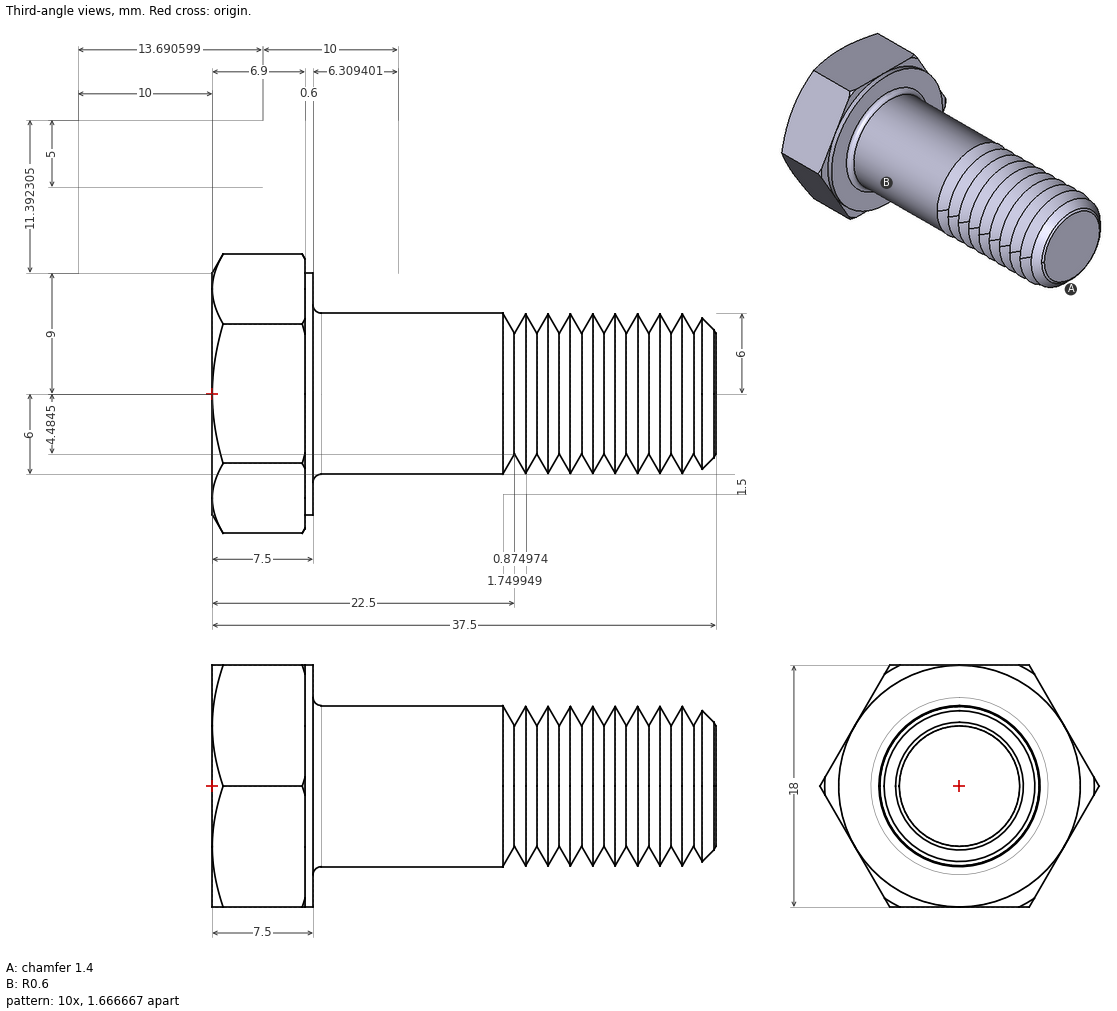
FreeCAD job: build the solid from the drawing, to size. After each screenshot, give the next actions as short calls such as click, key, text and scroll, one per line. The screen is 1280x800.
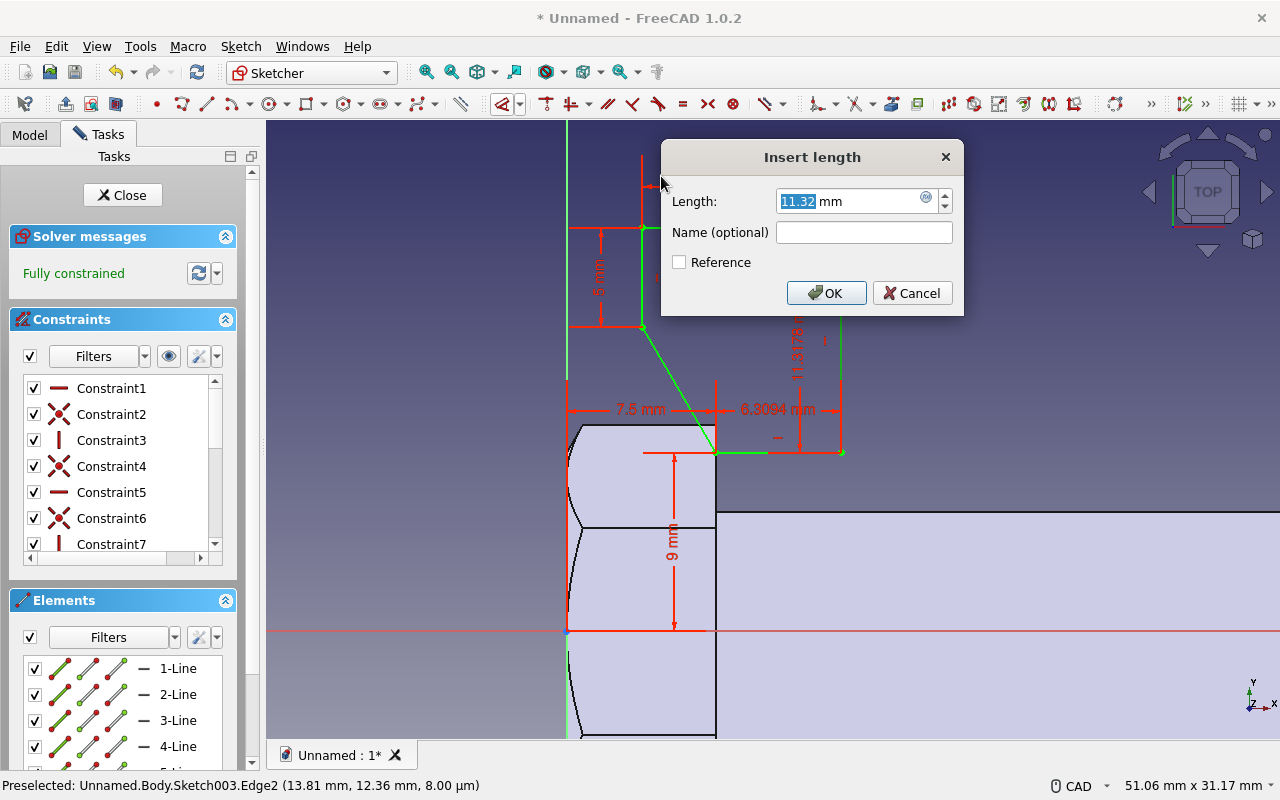
text(11.392305)
key(Return)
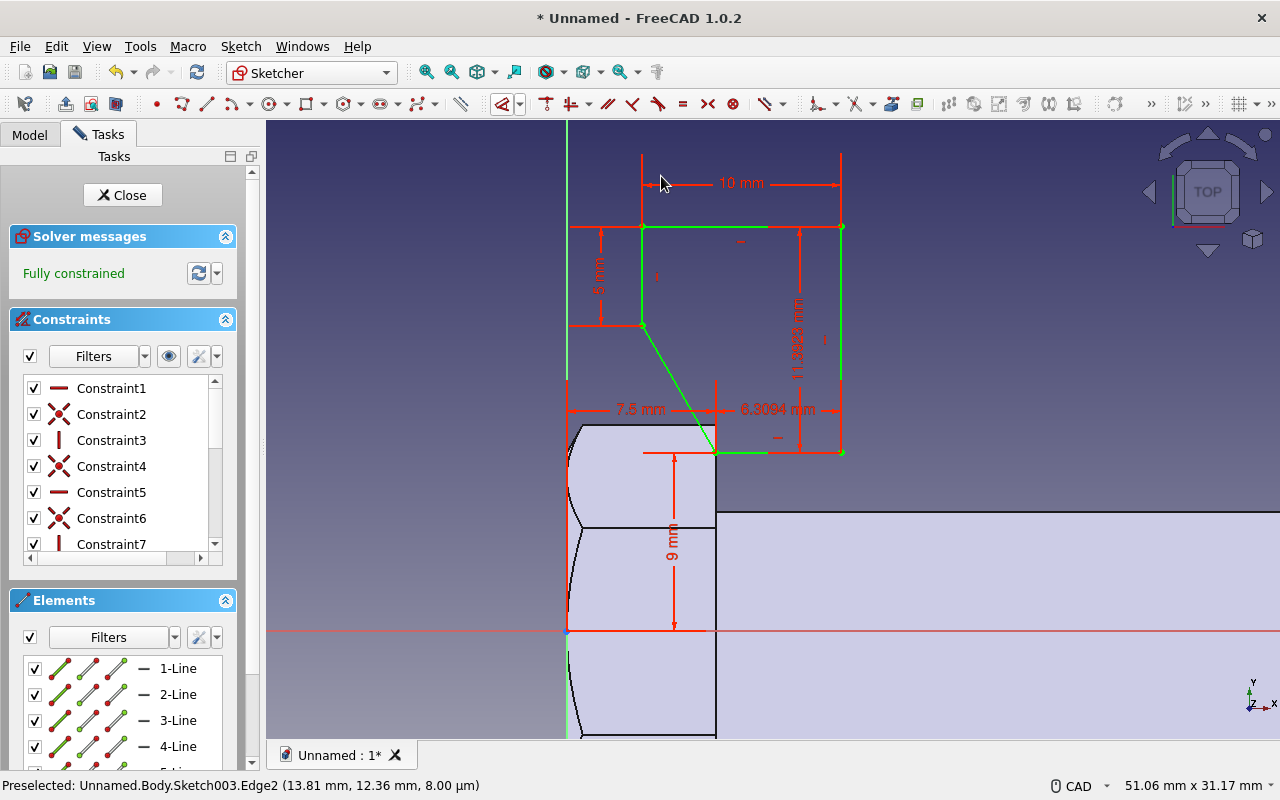
click(123, 195)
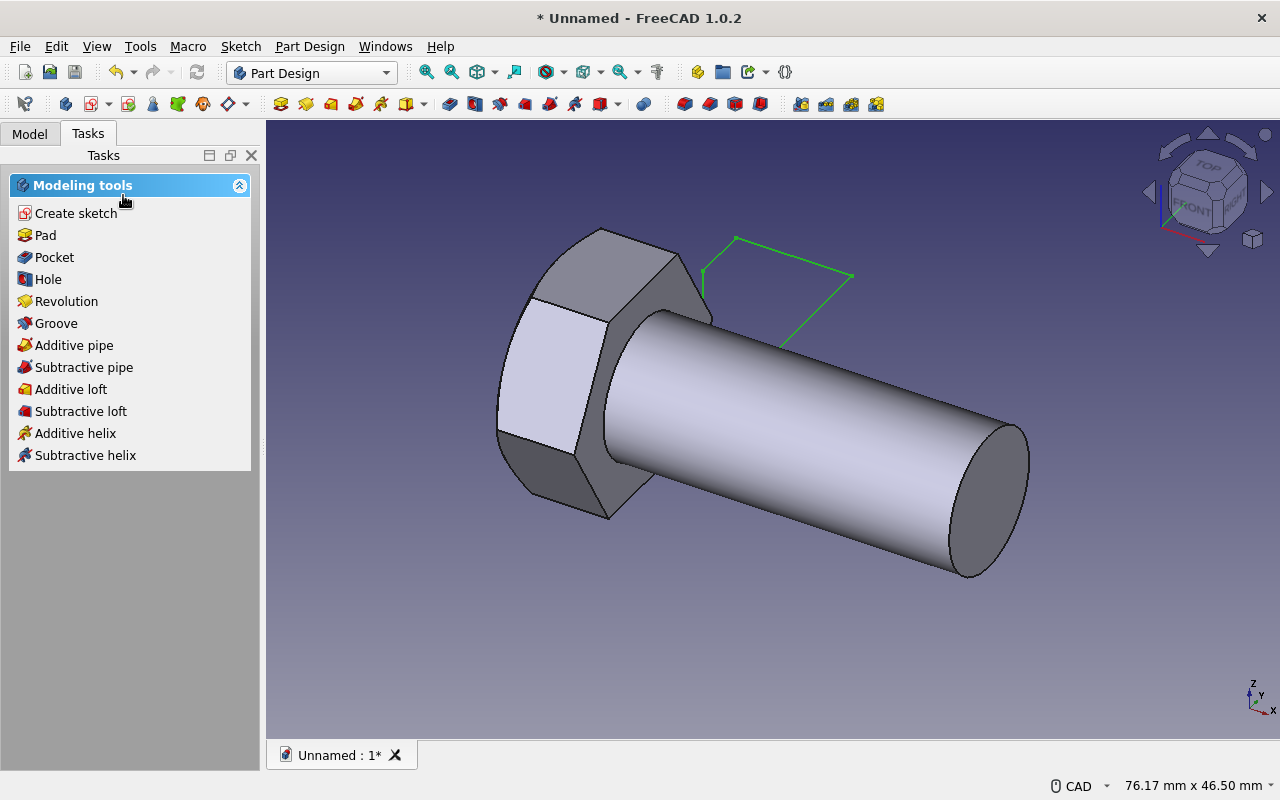
click(500, 104)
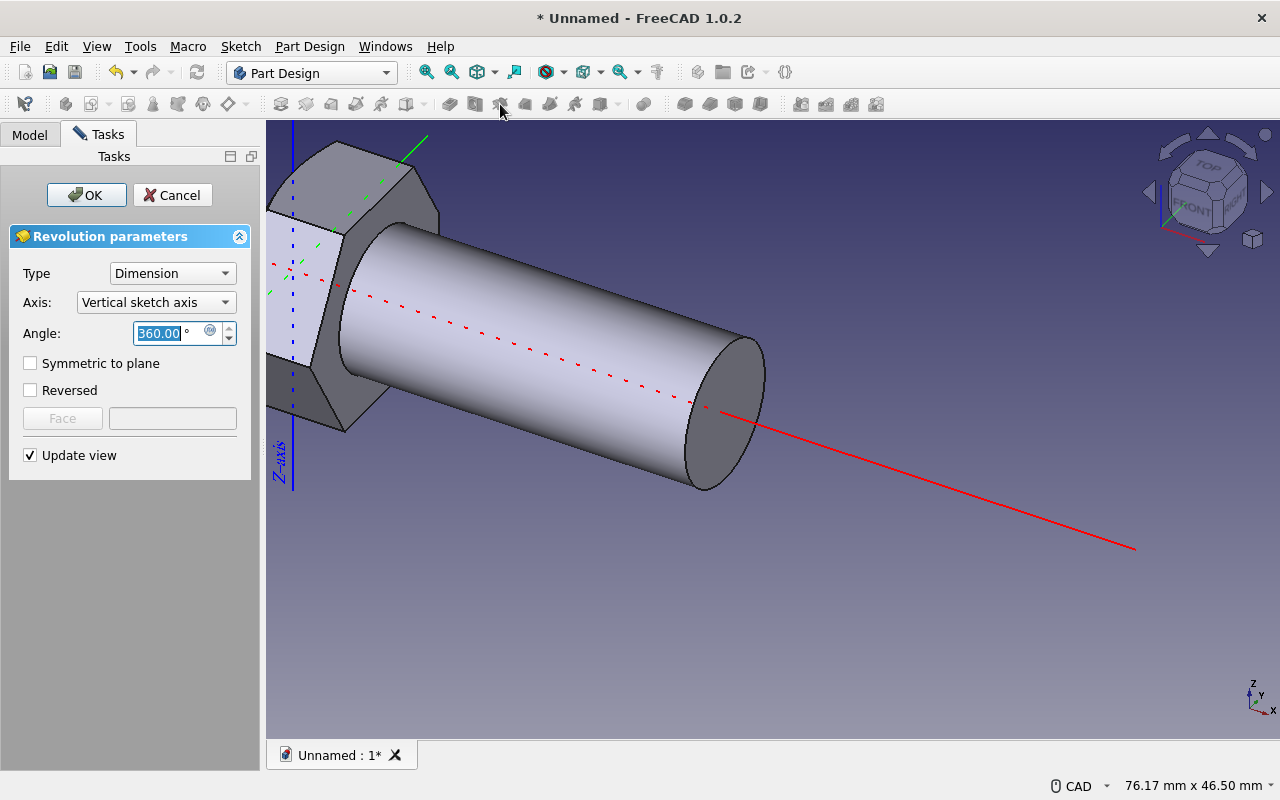
click(157, 302)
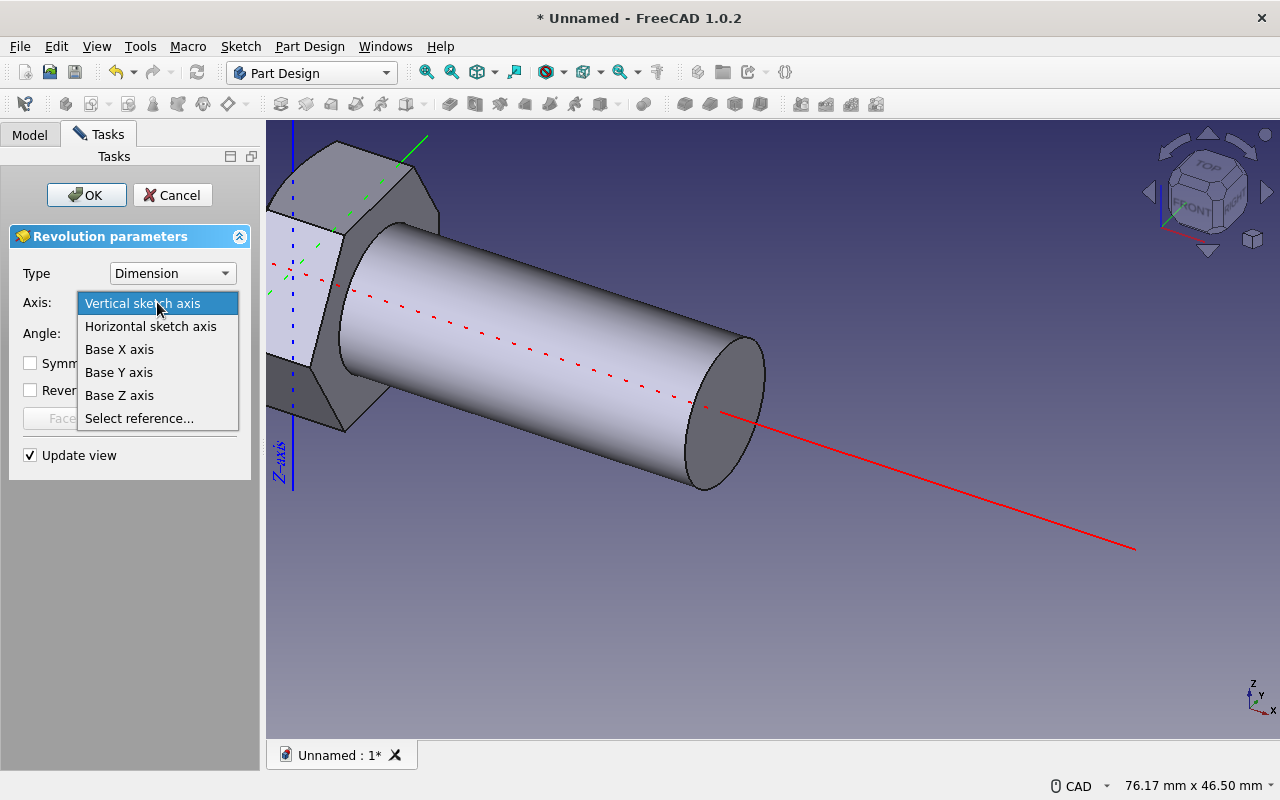
click(156, 326)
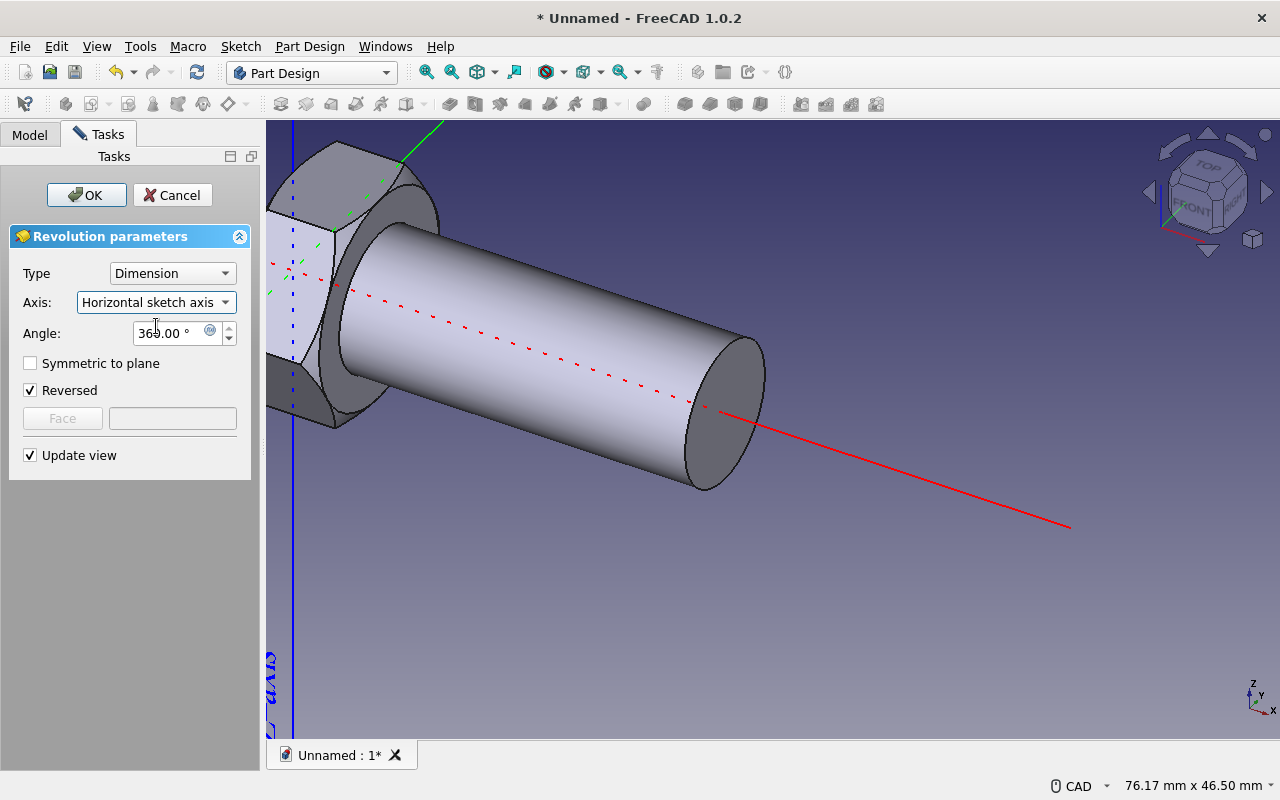
click(87, 195)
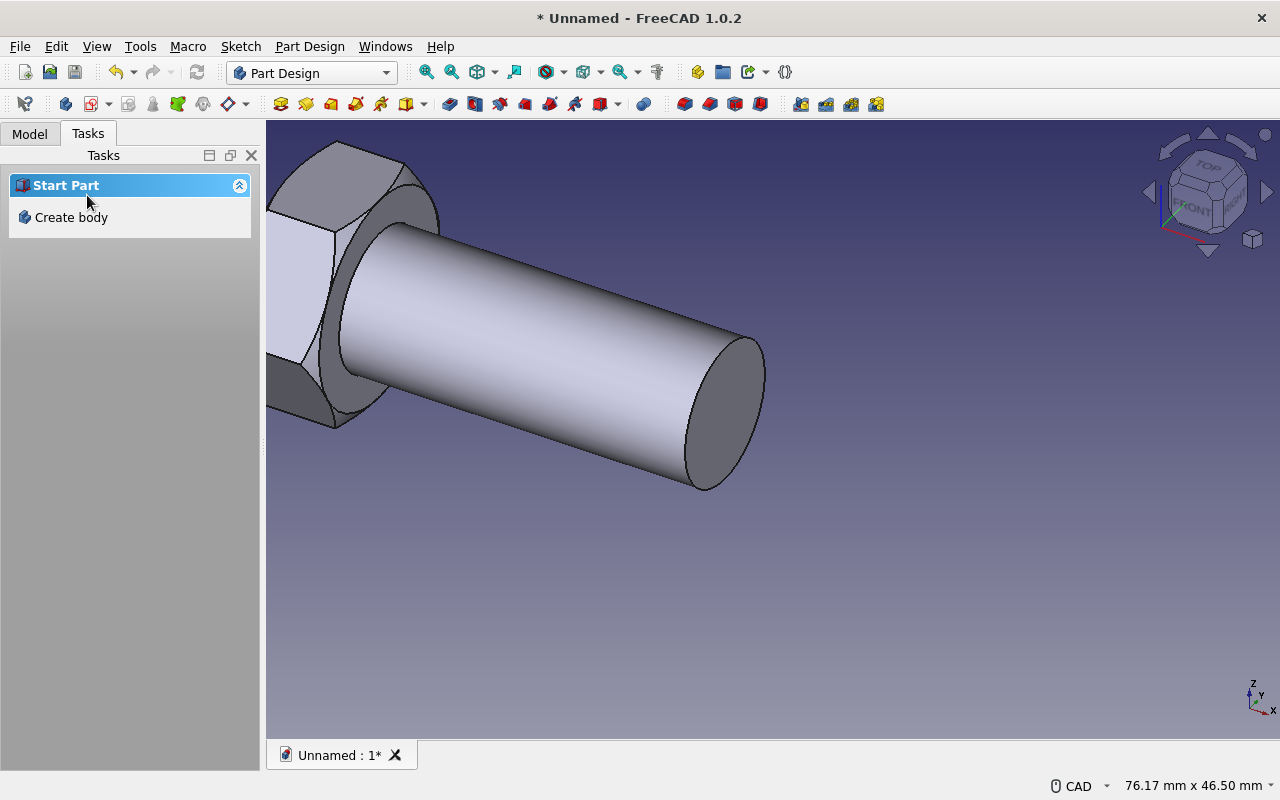
click(427, 72)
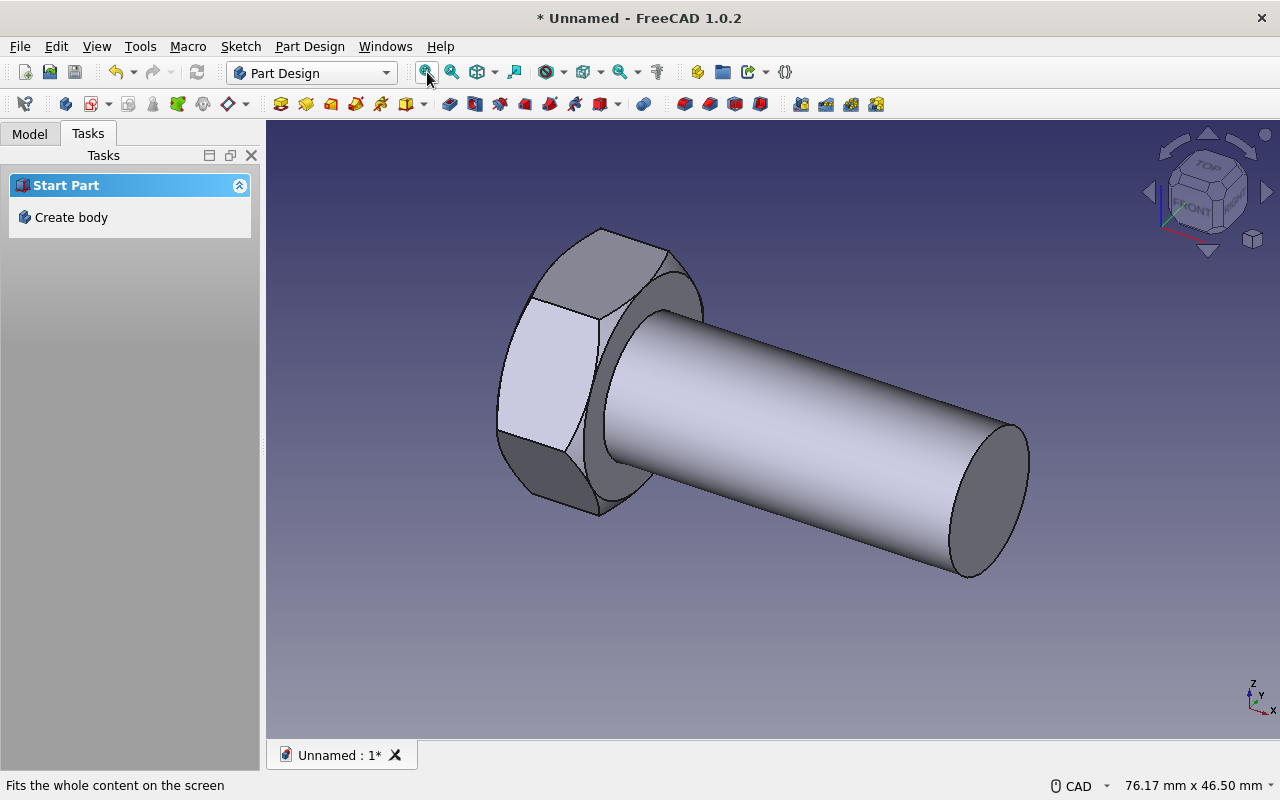
click(90, 104)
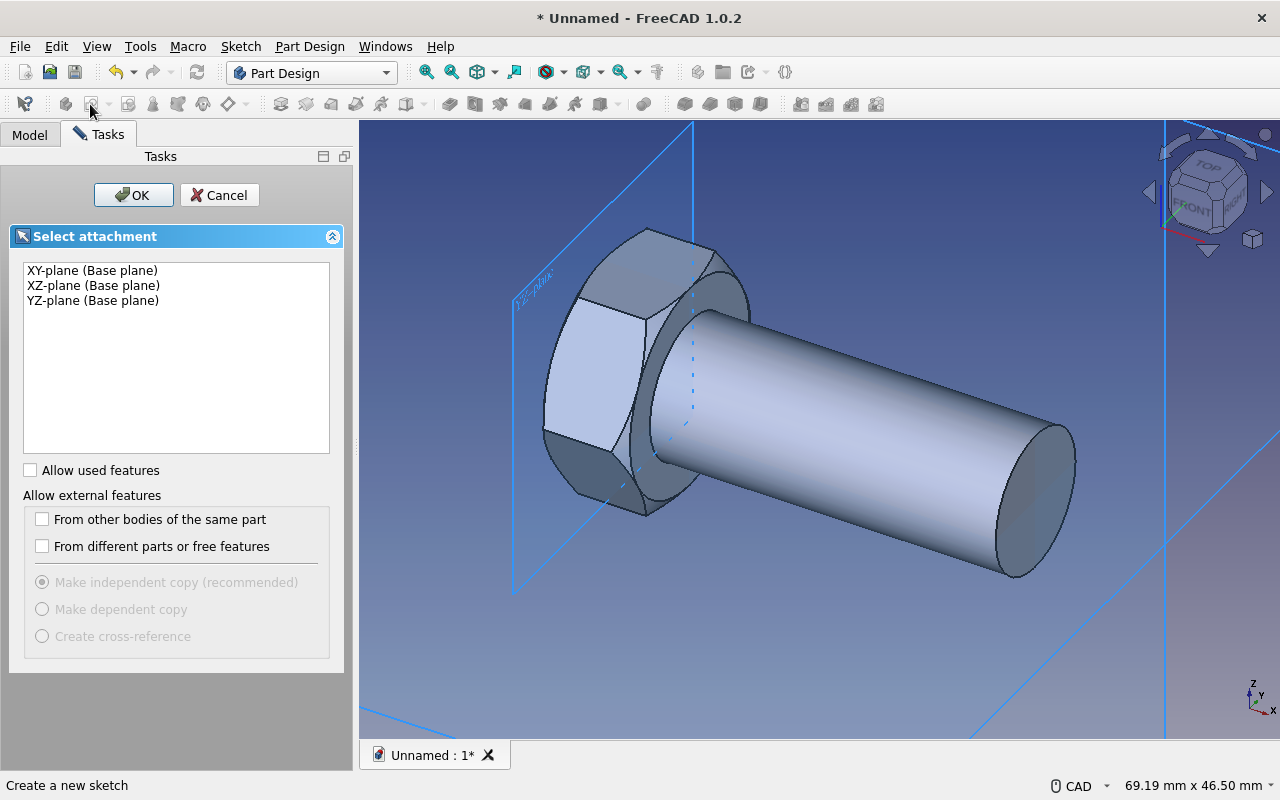
click(84, 270)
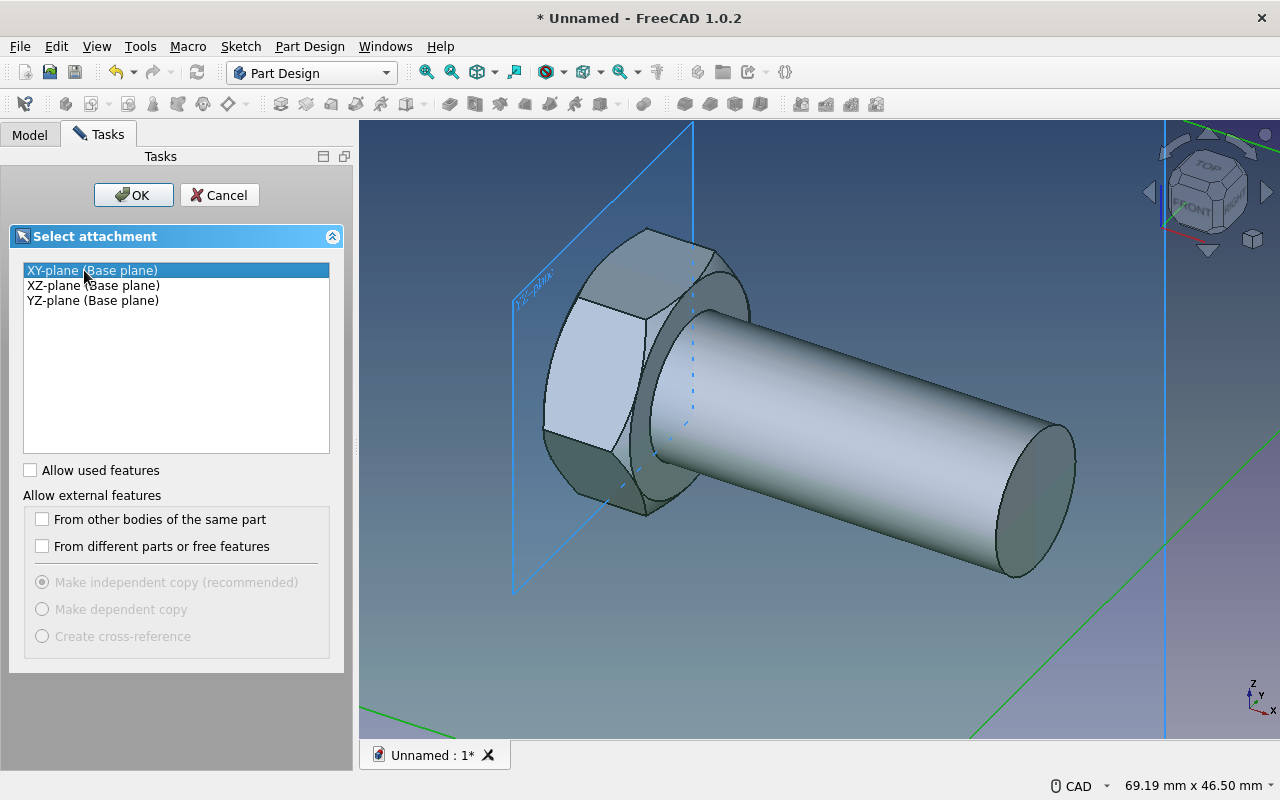
click(134, 195)